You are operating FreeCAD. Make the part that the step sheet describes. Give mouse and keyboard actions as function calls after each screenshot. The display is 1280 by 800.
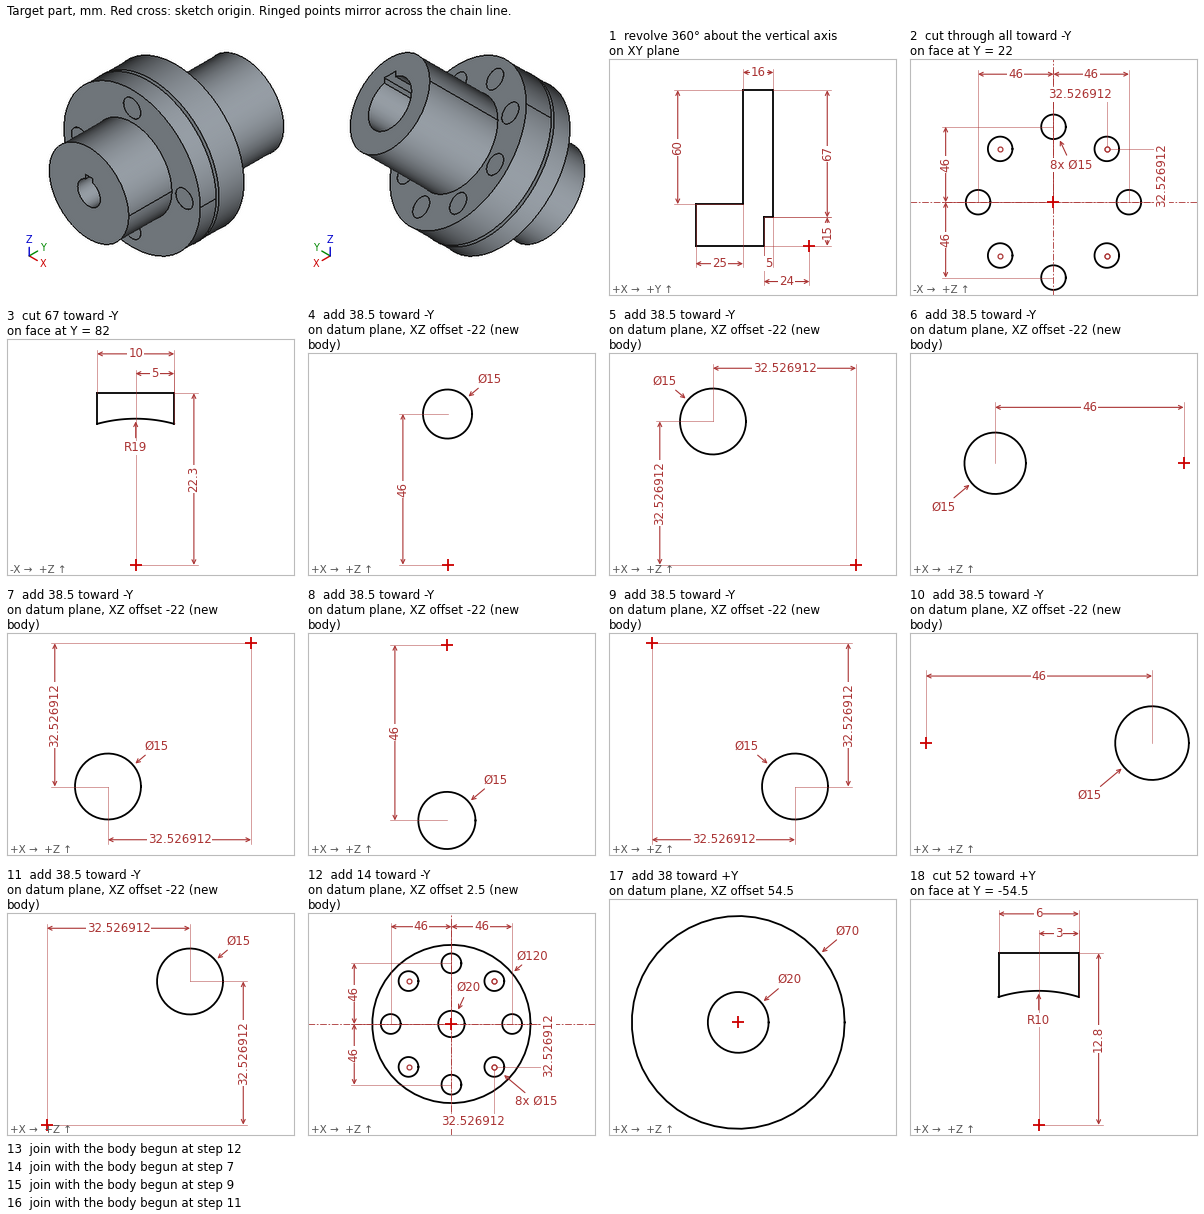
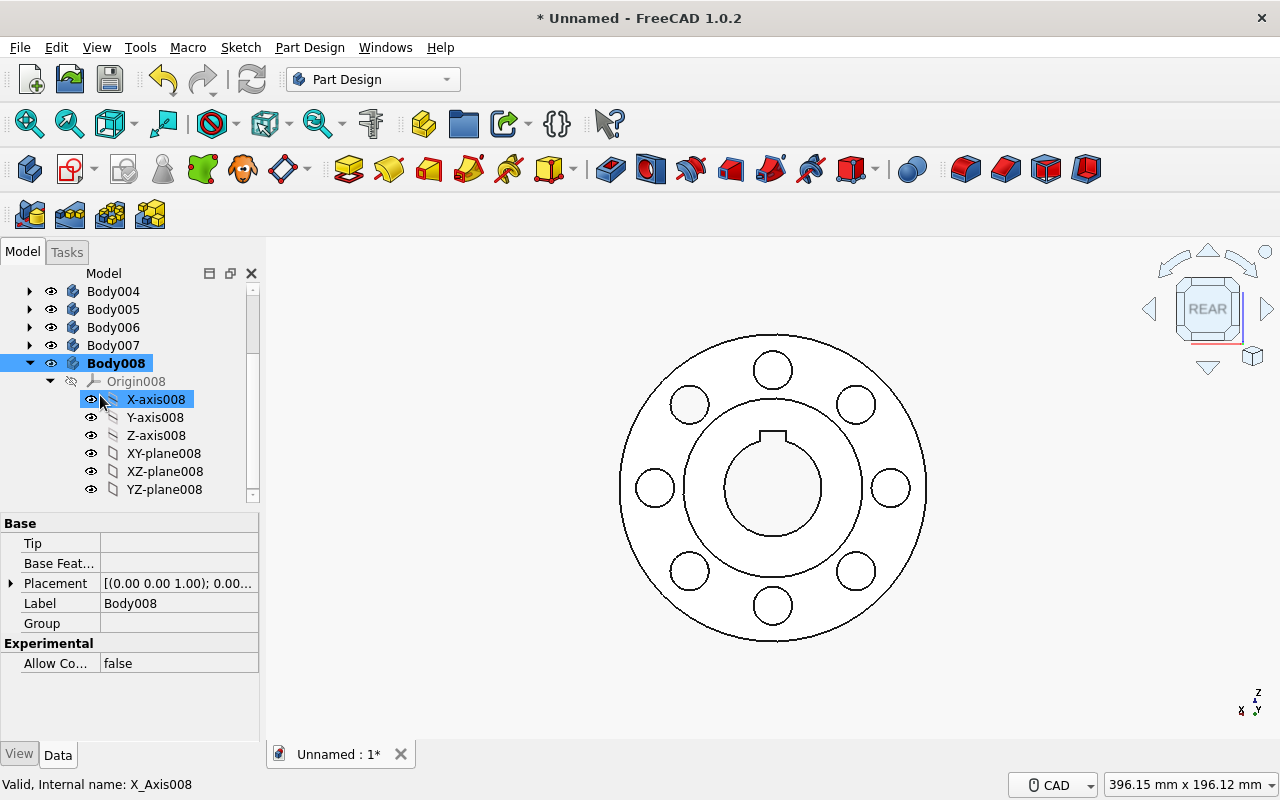
click(136, 471)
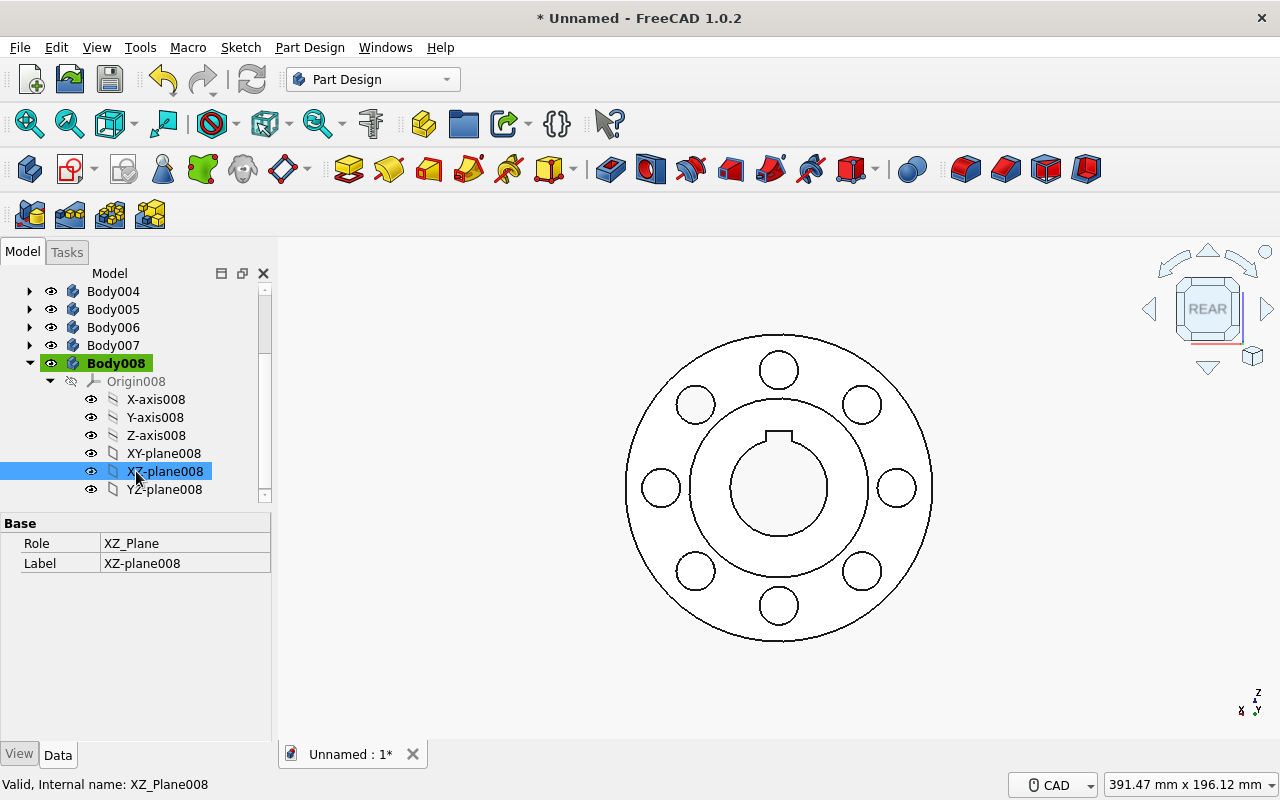
click(284, 170)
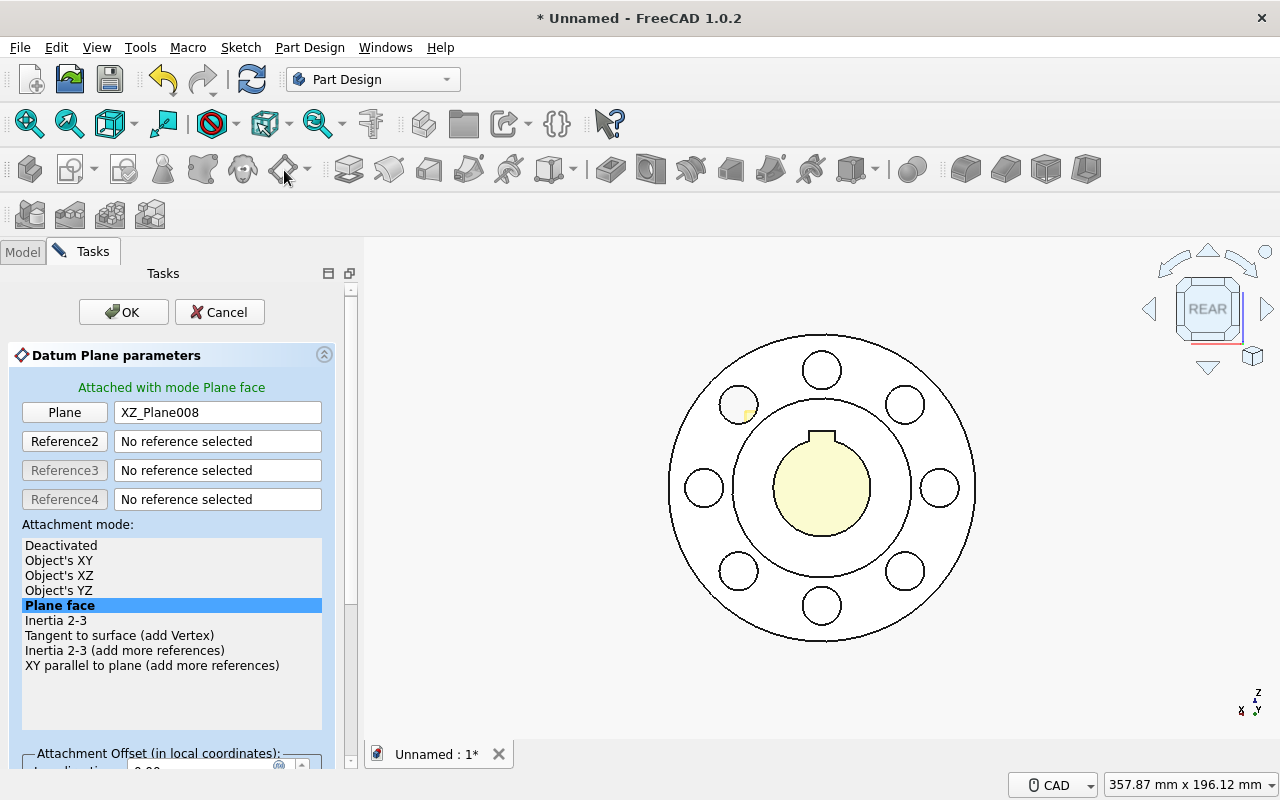
scroll(351, 526, down, 3)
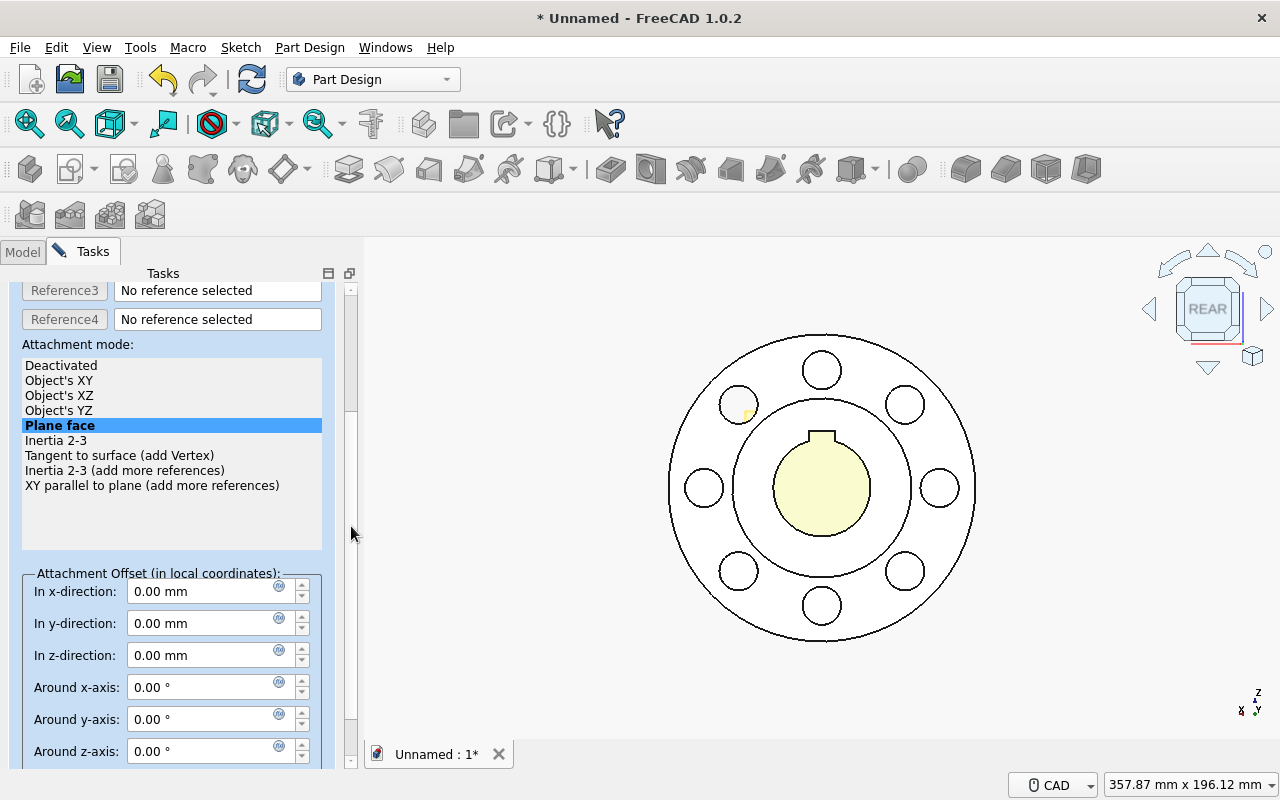
triple_click(210, 655)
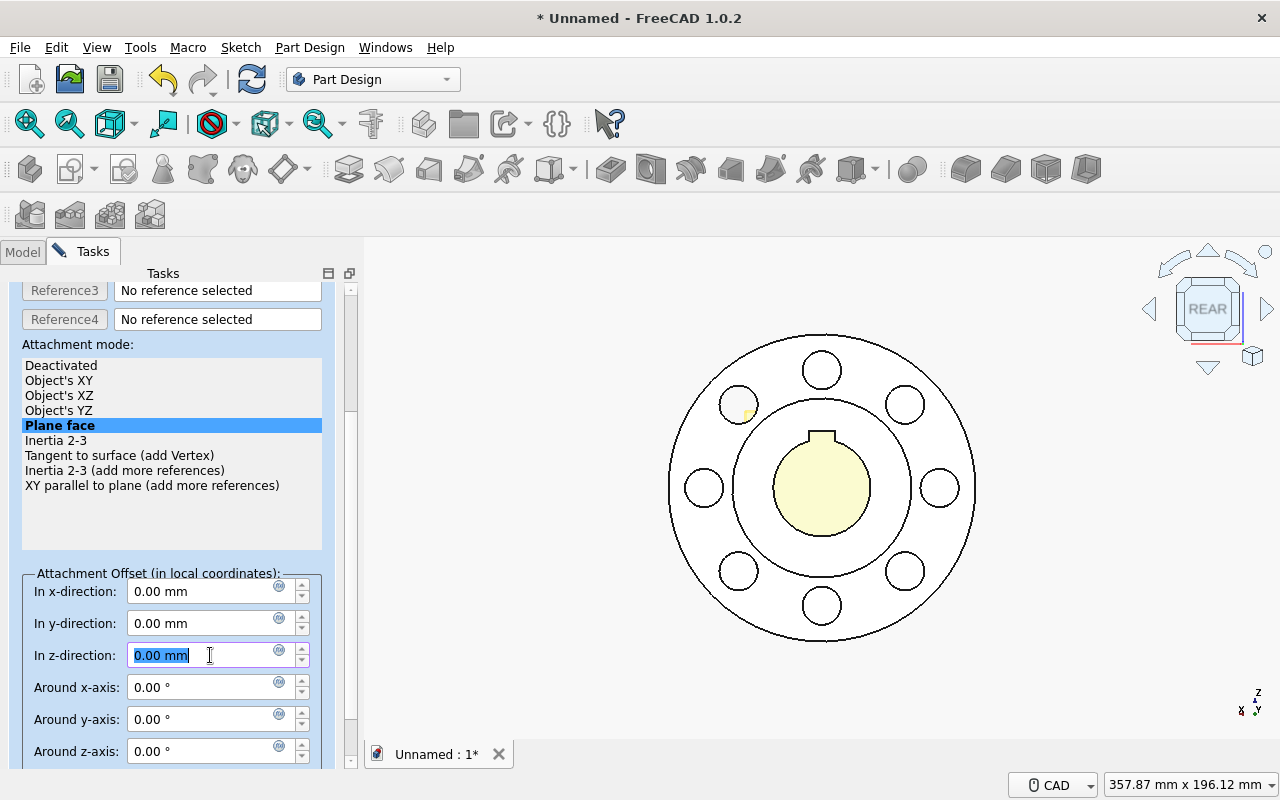
text(-22)
key(Tab)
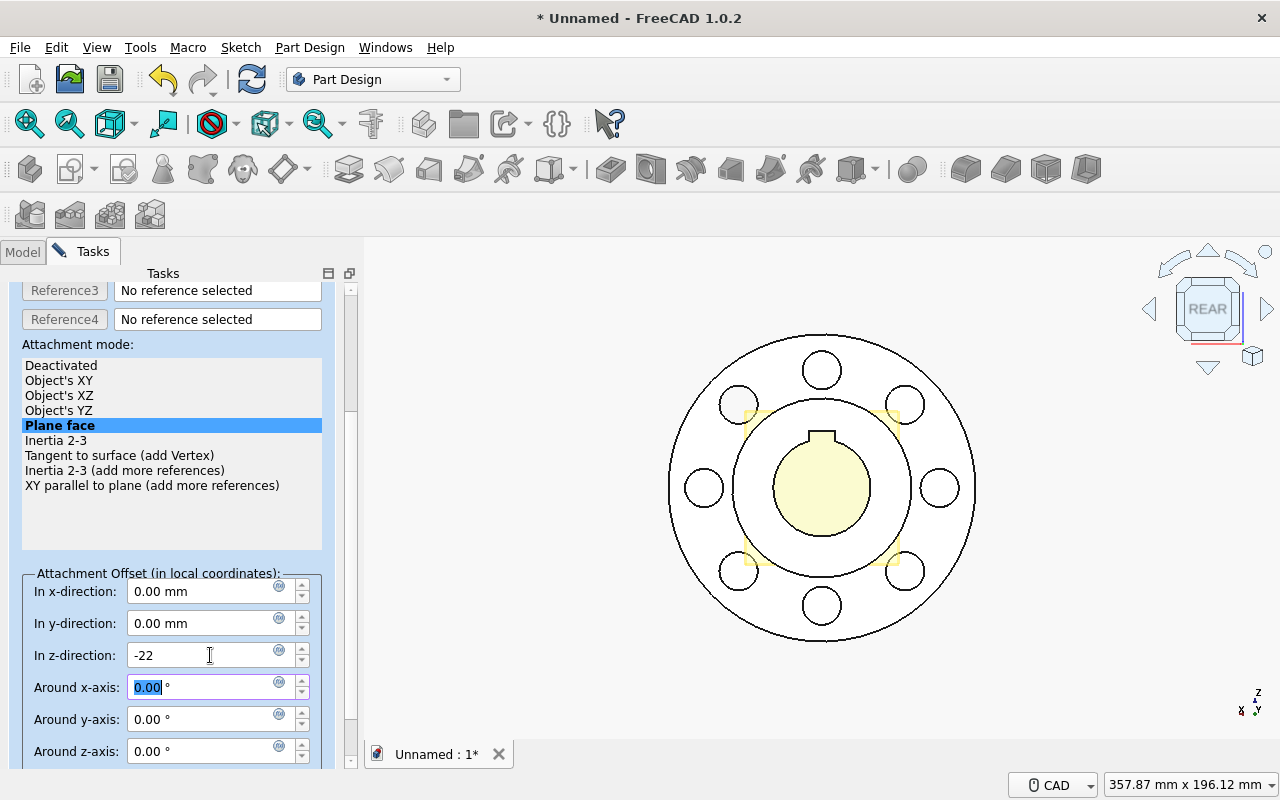
scroll(351, 526, up, 4)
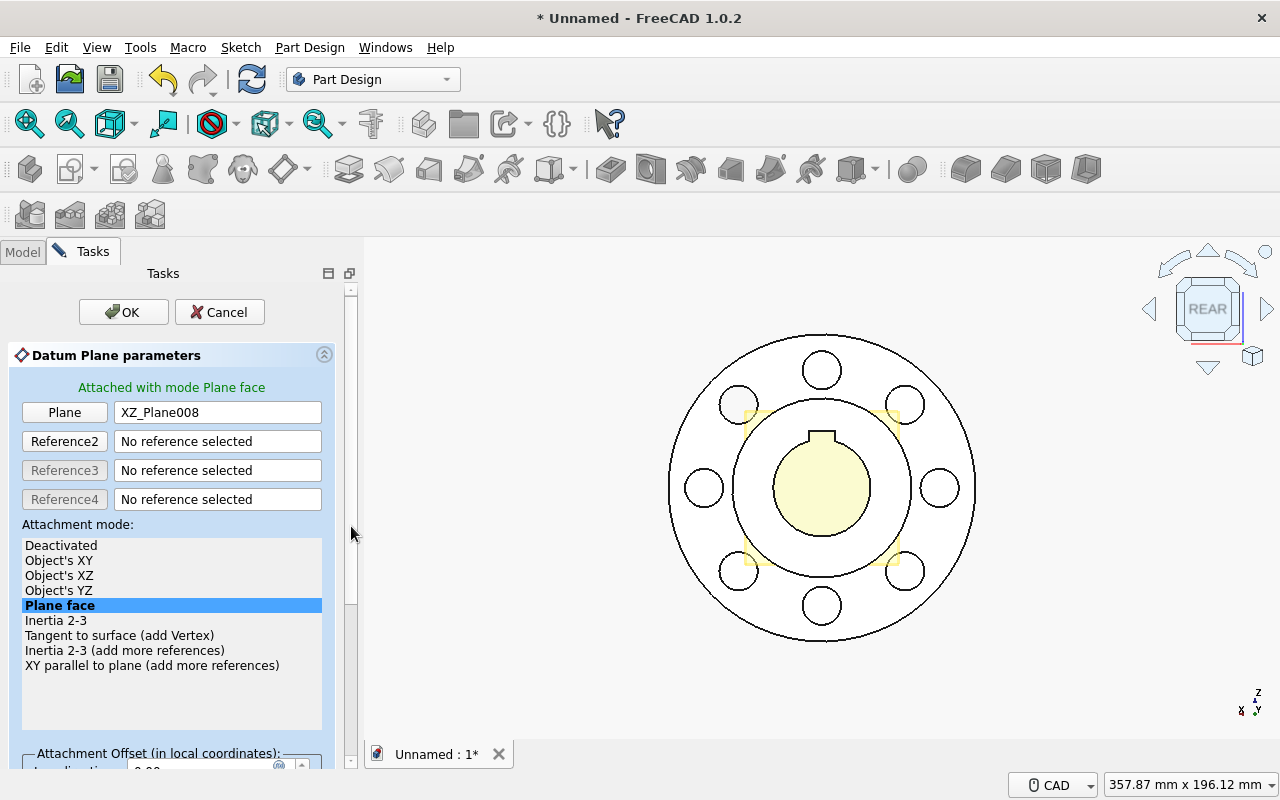
click(124, 312)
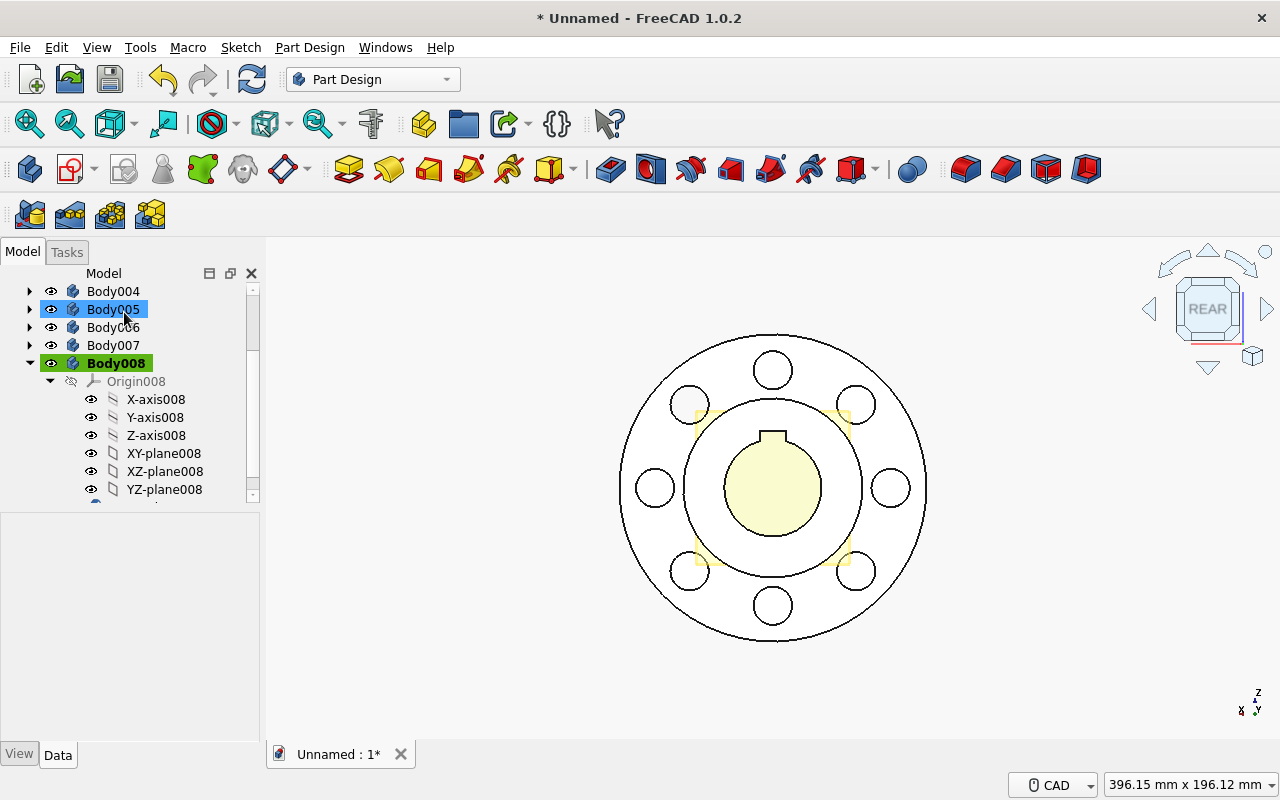
scroll(120, 395, down, 3)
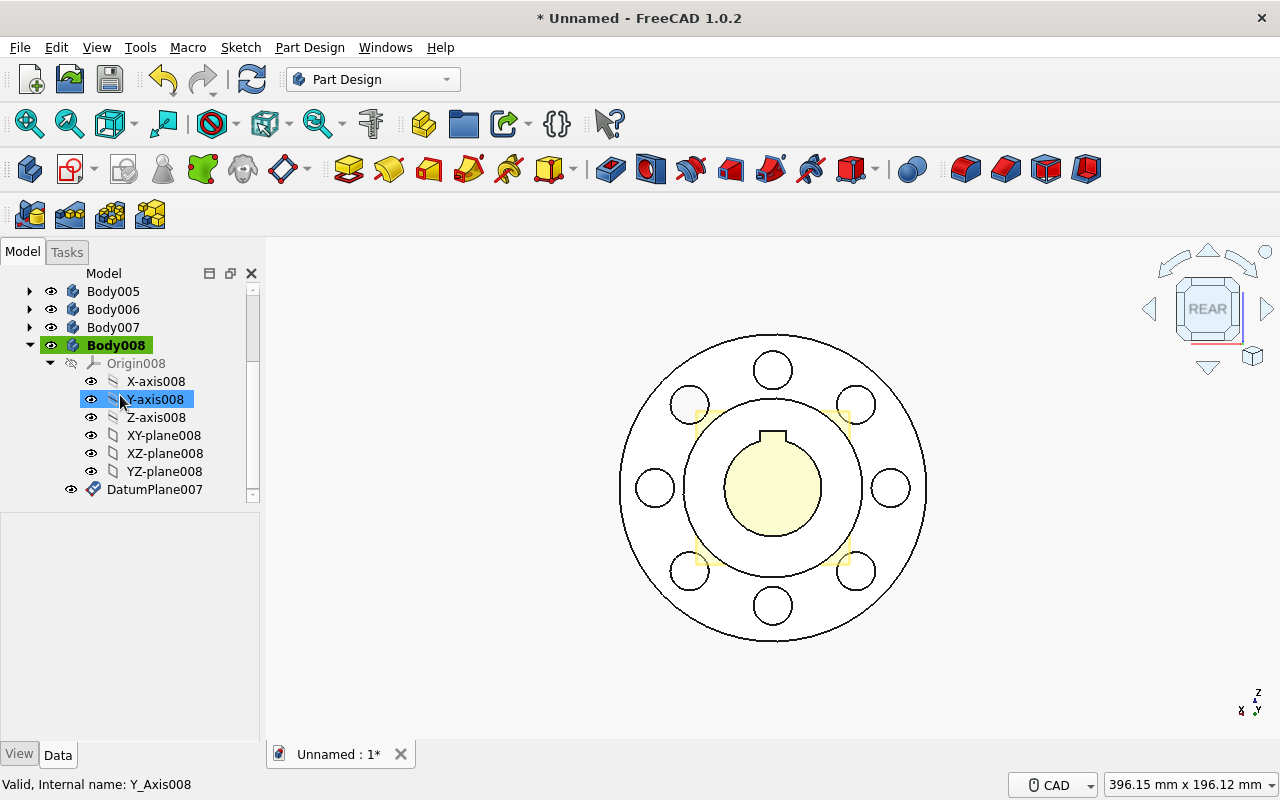
click(116, 489)